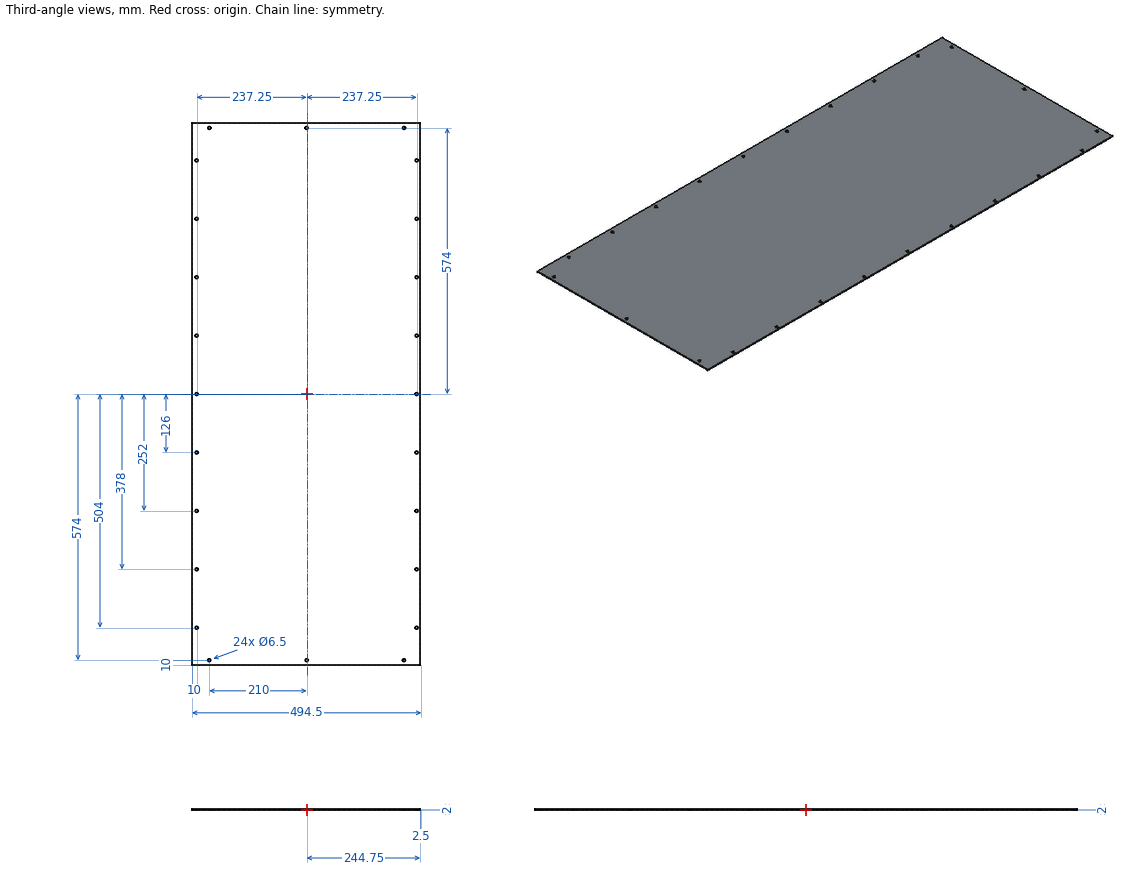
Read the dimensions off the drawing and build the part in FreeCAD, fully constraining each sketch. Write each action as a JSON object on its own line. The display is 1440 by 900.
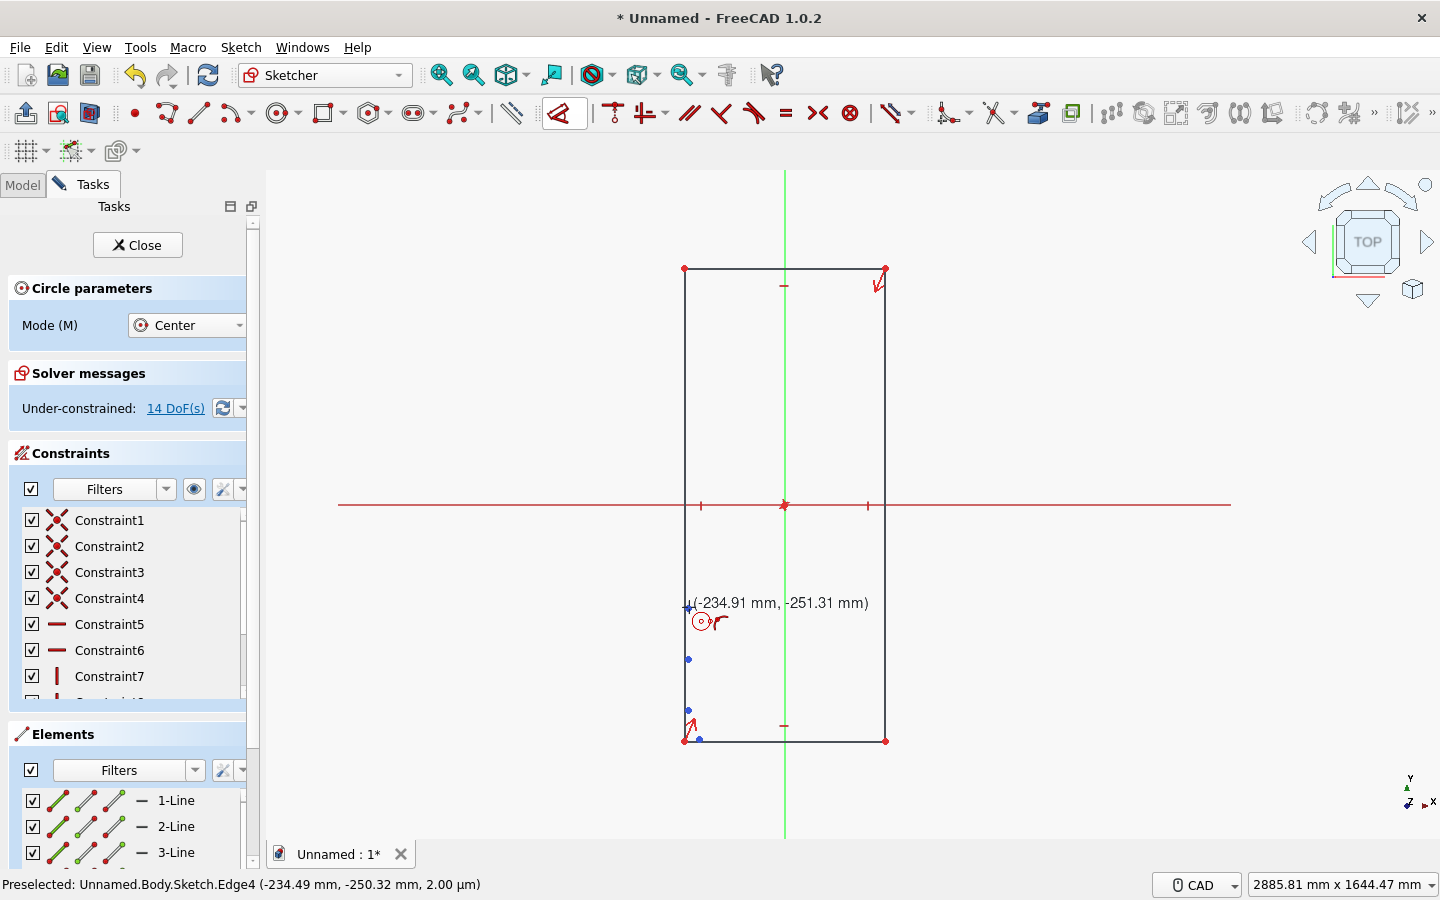
{"action": "scroll", "coordinate": [688, 557], "scroll_direction": "up", "scroll_amount": 15}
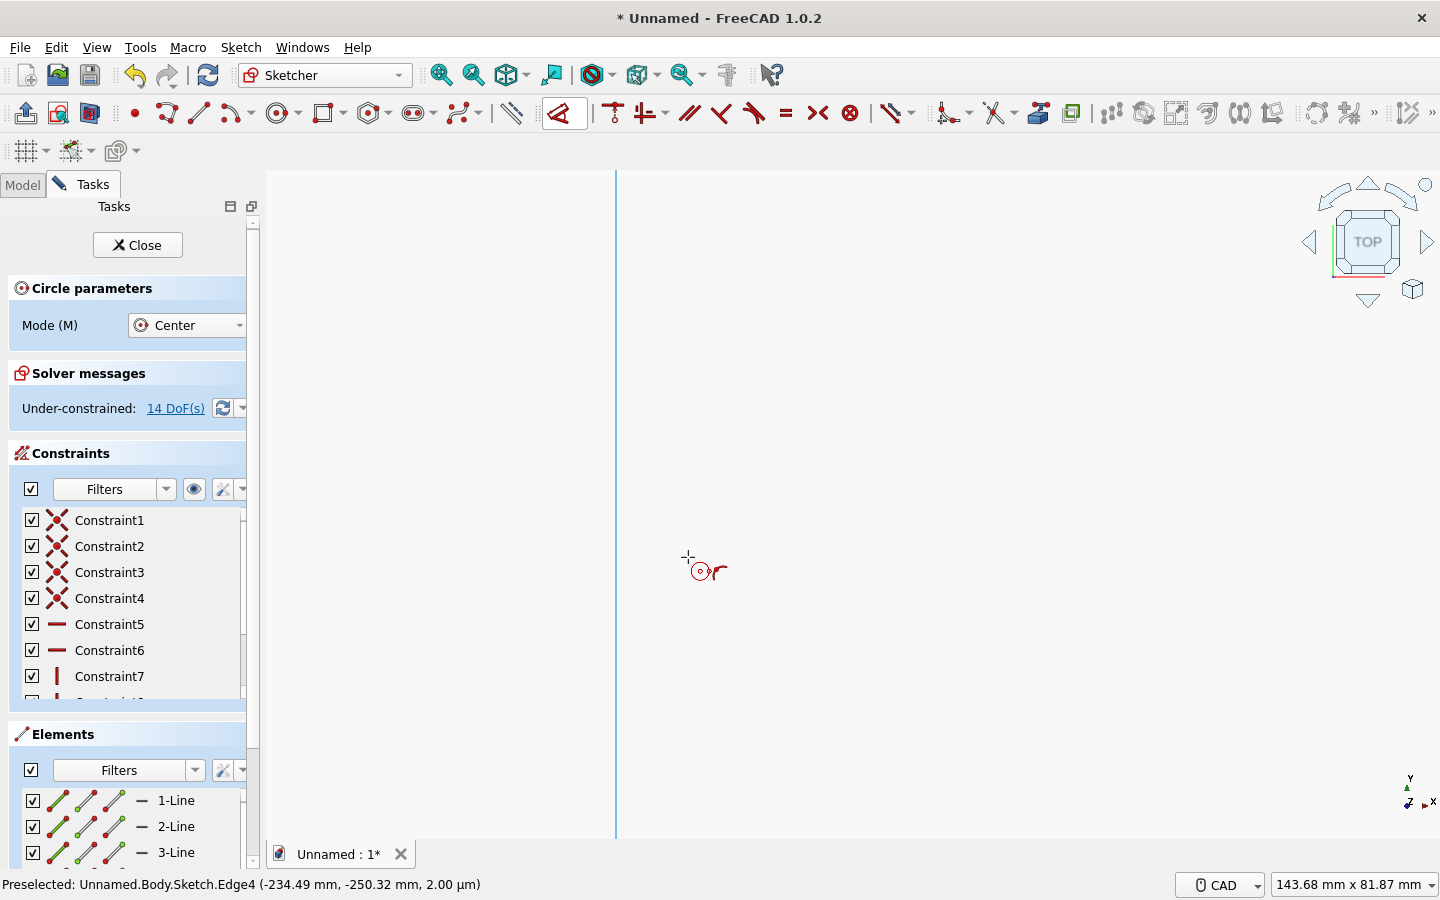
{"action": "scroll", "coordinate": [688, 557], "scroll_direction": "down", "scroll_amount": 15}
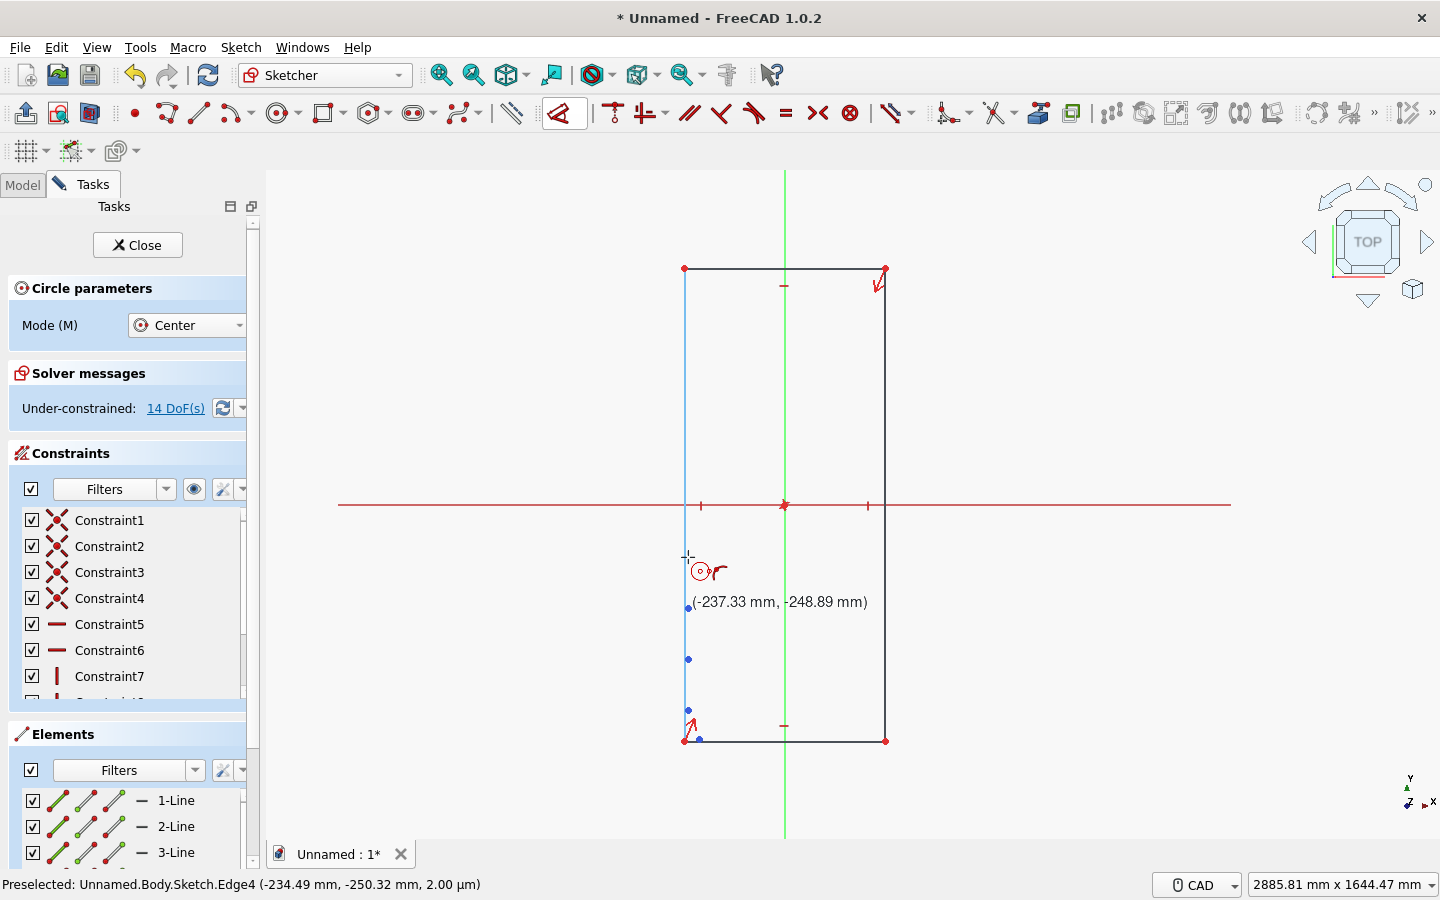
{"action": "scroll", "coordinate": [688, 557], "scroll_direction": "up", "scroll_amount": 7}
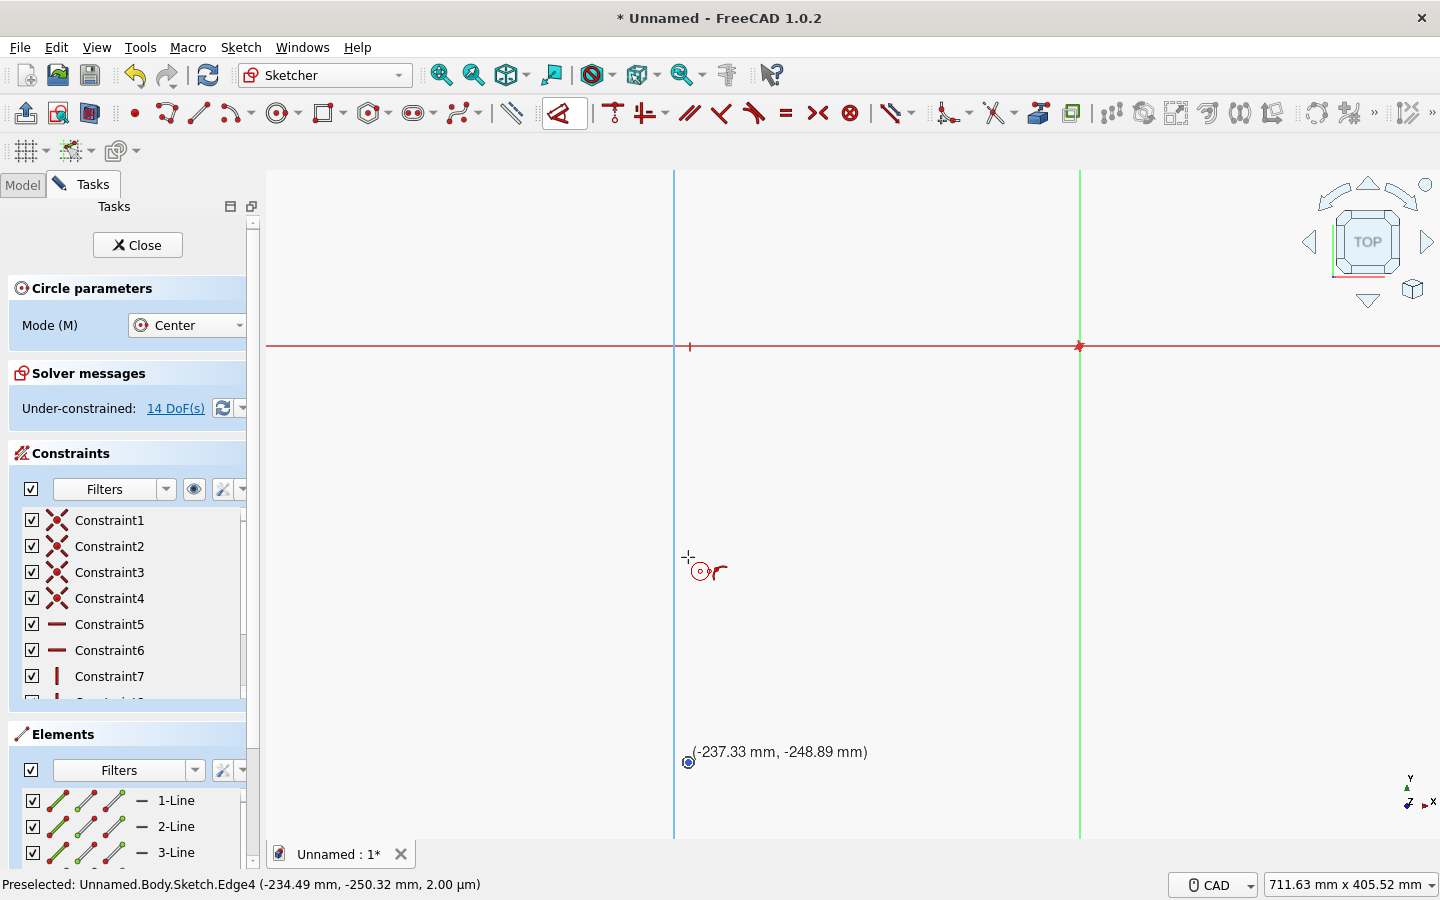
{"action": "left_click", "coordinate": [688, 554]}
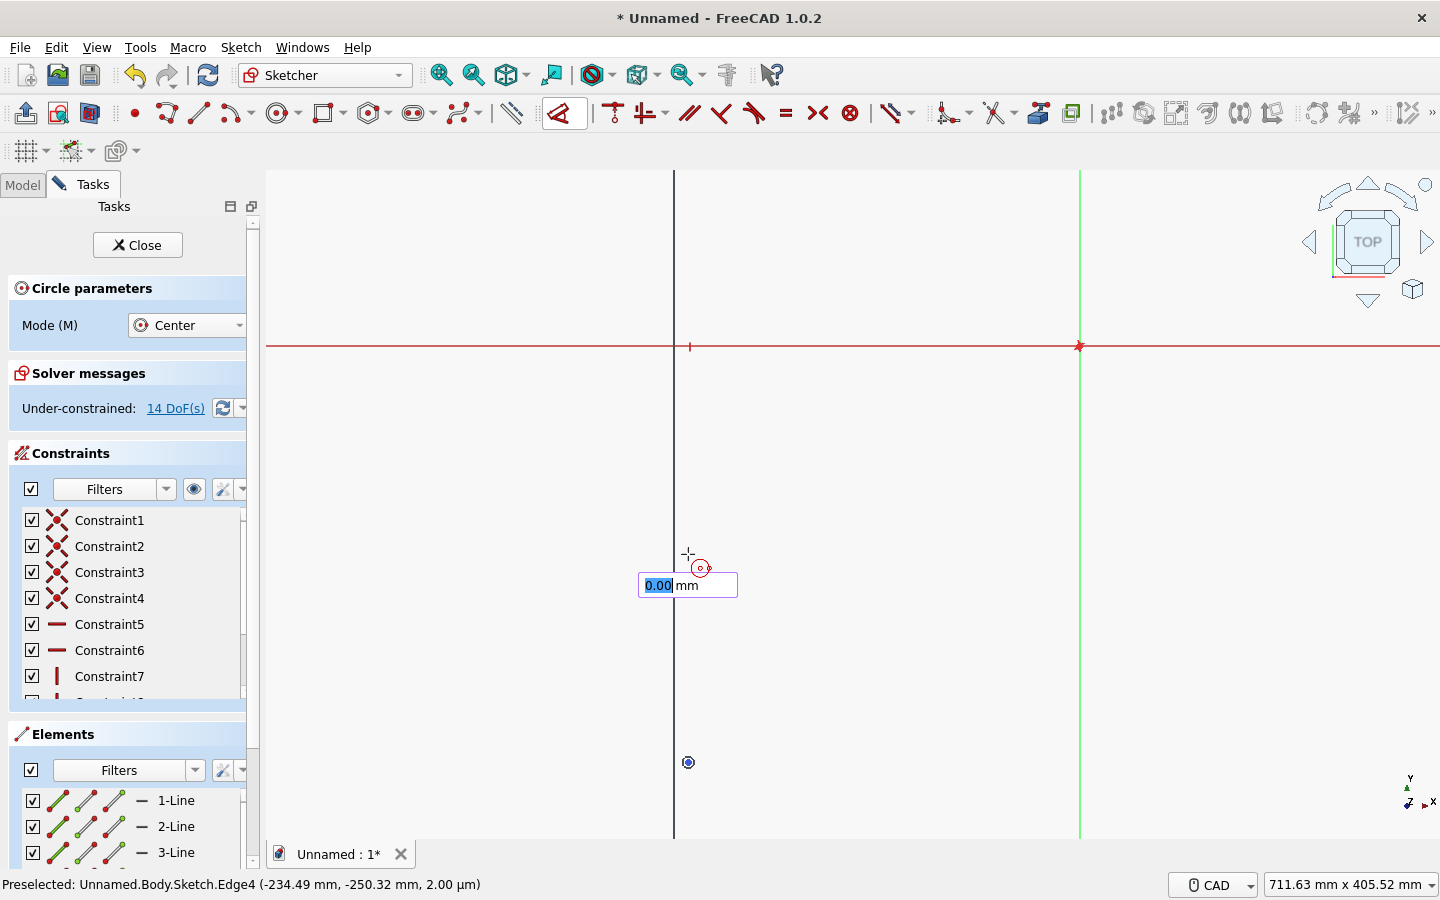
{"action": "scroll", "coordinate": [692, 550], "scroll_direction": "up", "scroll_amount": 6}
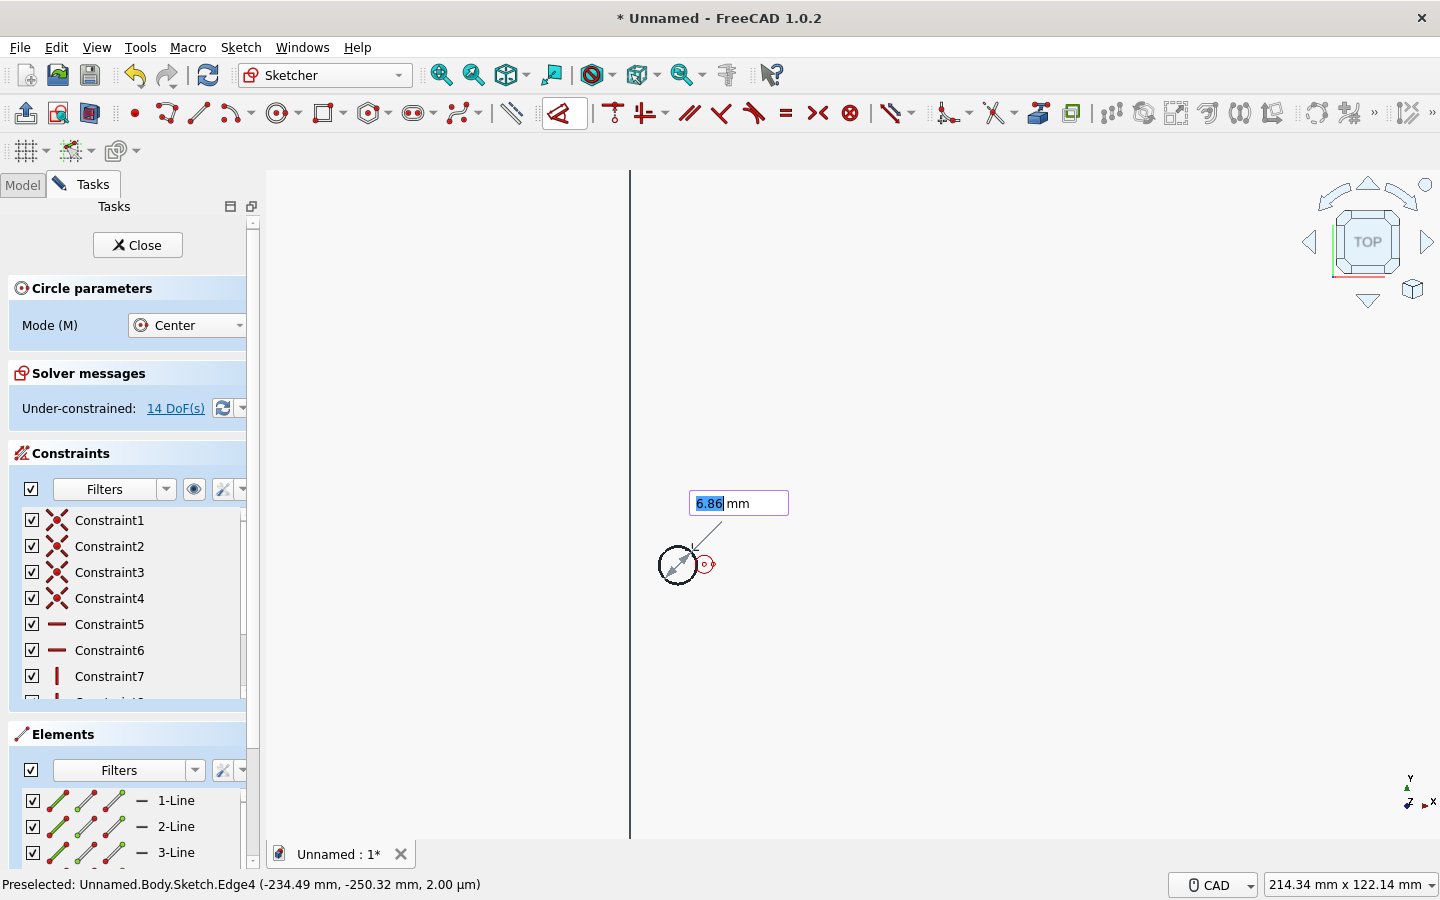
{"action": "left_click", "coordinate": [692, 549]}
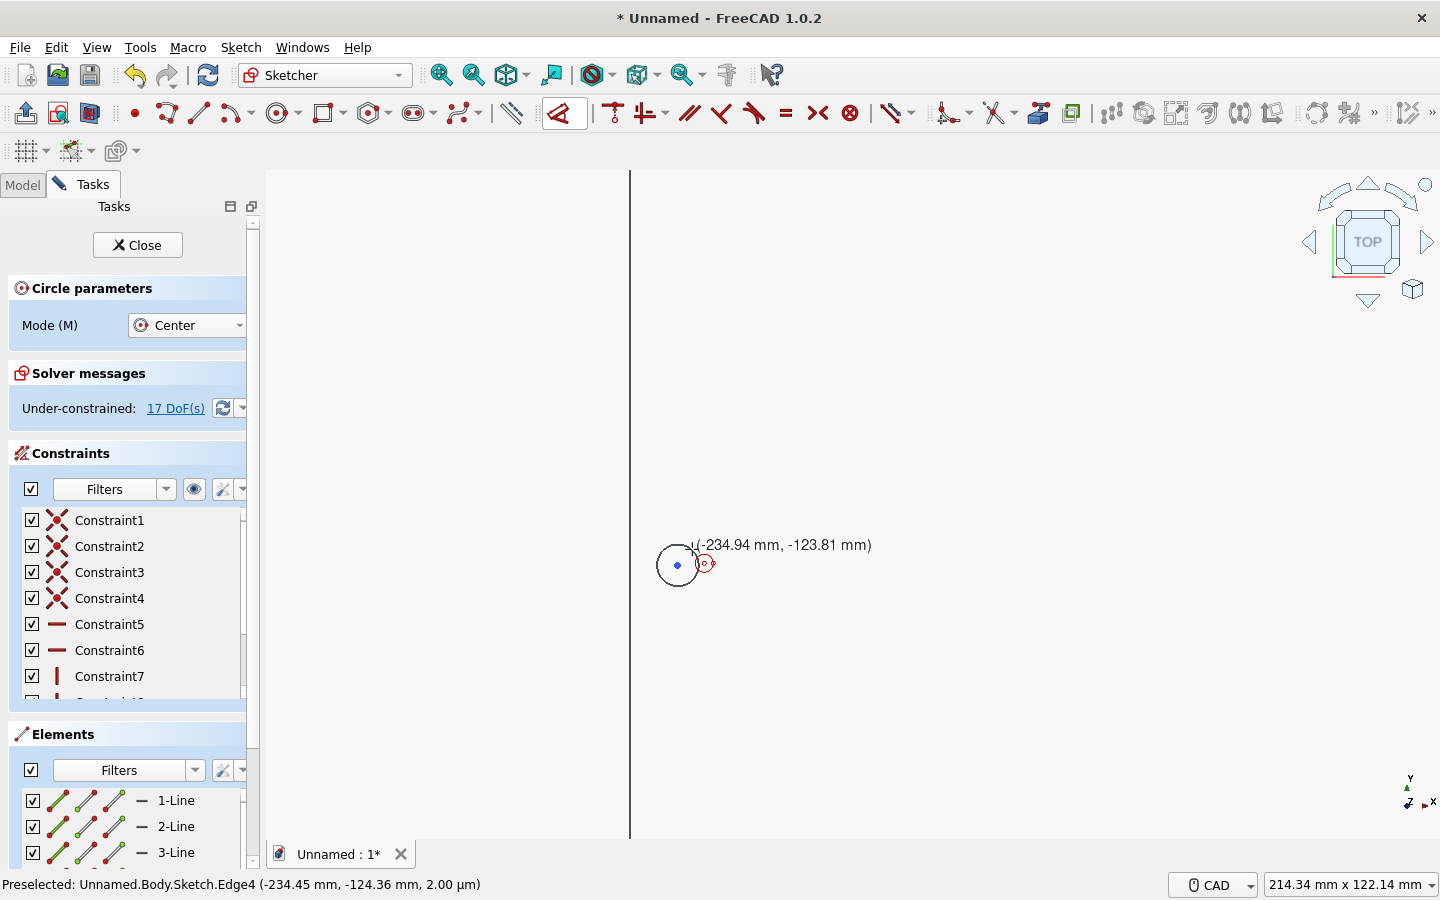
{"action": "scroll", "coordinate": [689, 555], "scroll_direction": "down", "scroll_amount": 13}